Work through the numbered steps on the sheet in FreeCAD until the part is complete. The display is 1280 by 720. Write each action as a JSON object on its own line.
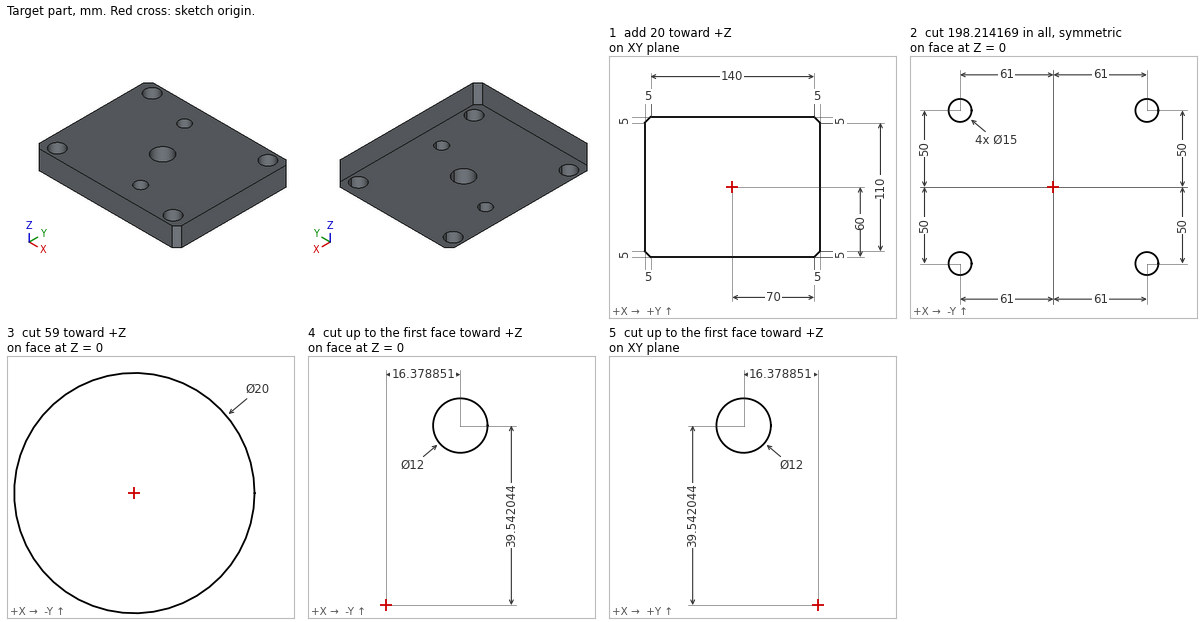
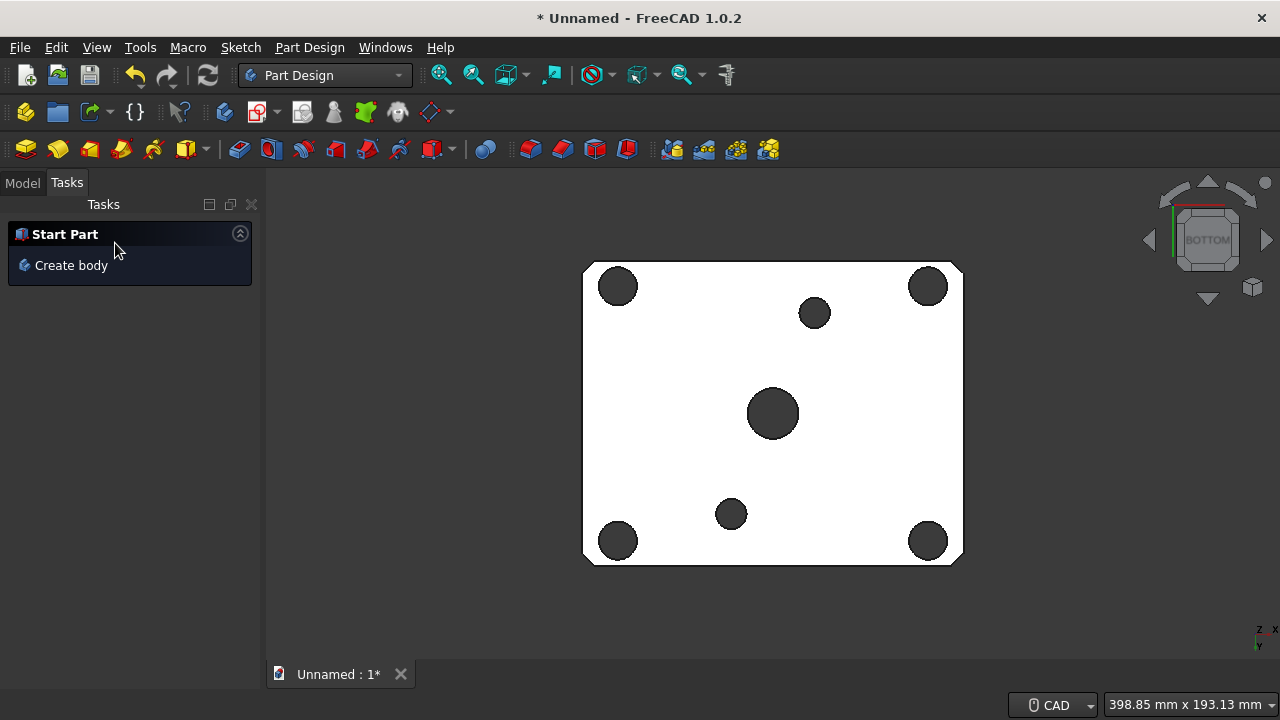
{"action": "key", "text": "0"}